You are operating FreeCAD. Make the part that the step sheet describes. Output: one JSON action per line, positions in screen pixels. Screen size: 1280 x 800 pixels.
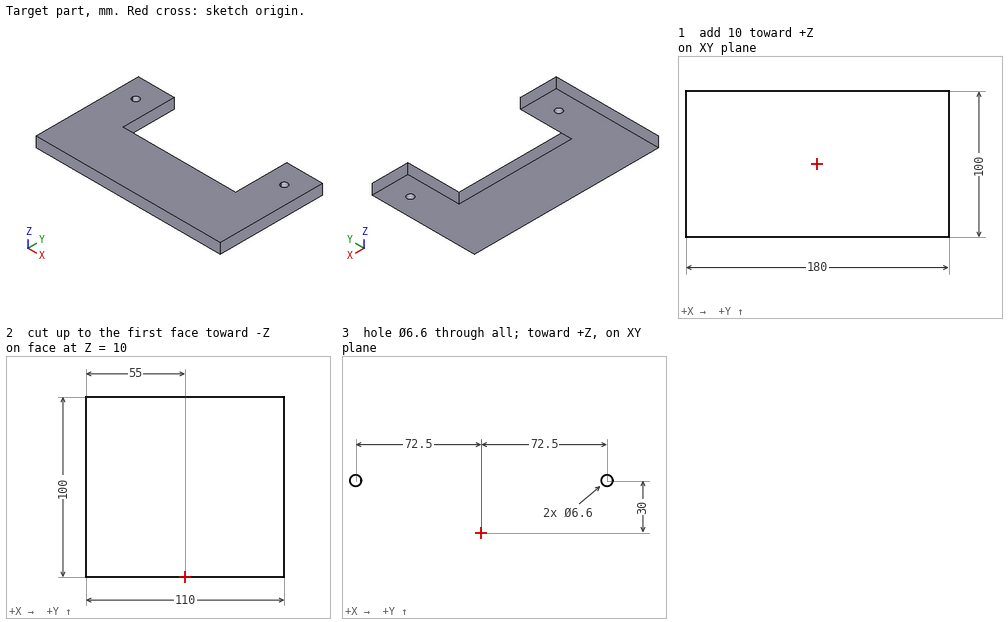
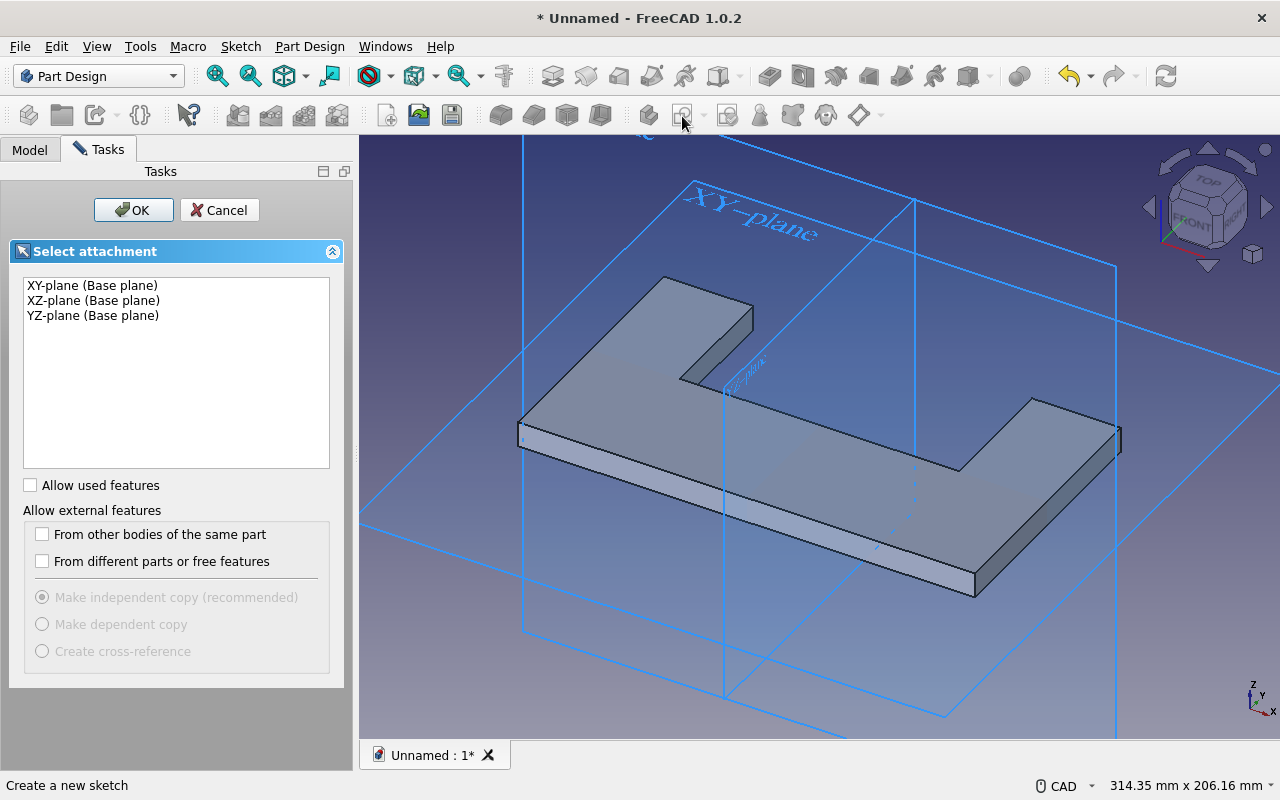
{"action": "left_click", "coordinate": [84, 286]}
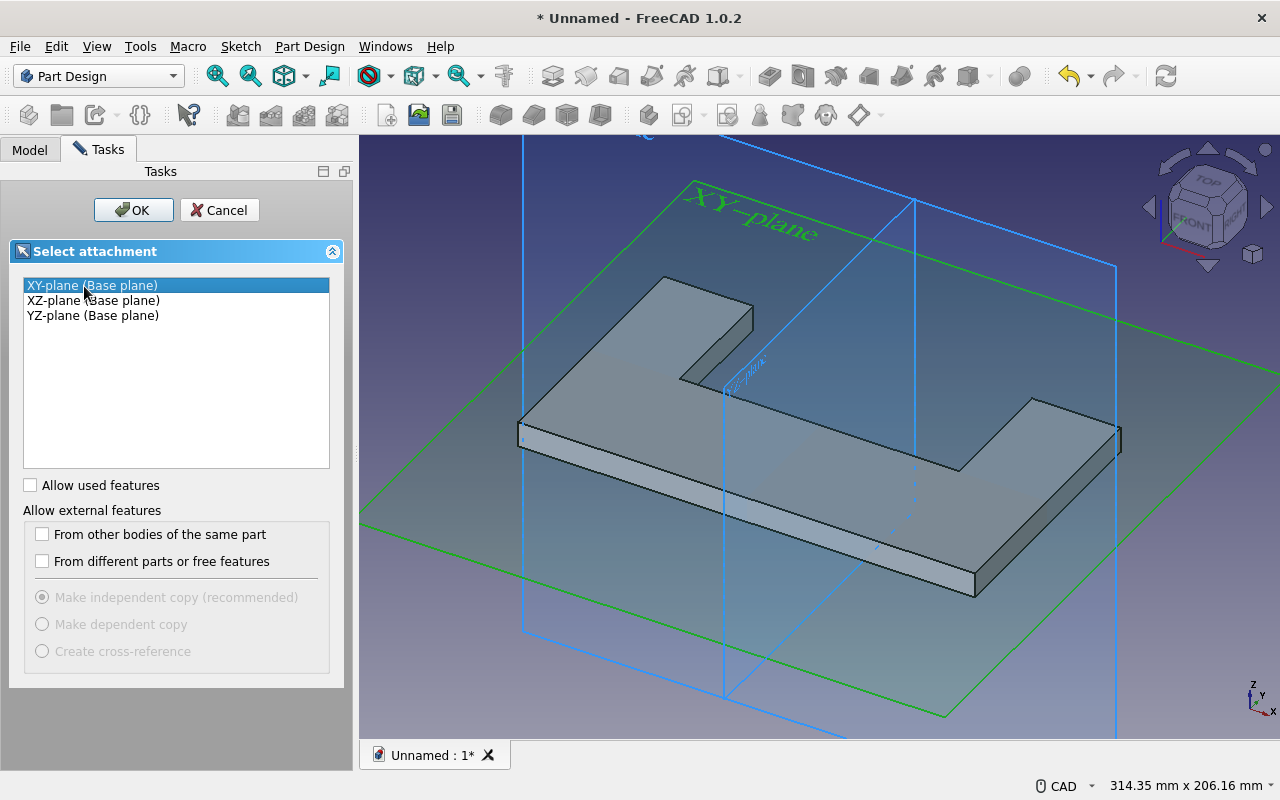
{"action": "left_click", "coordinate": [134, 210]}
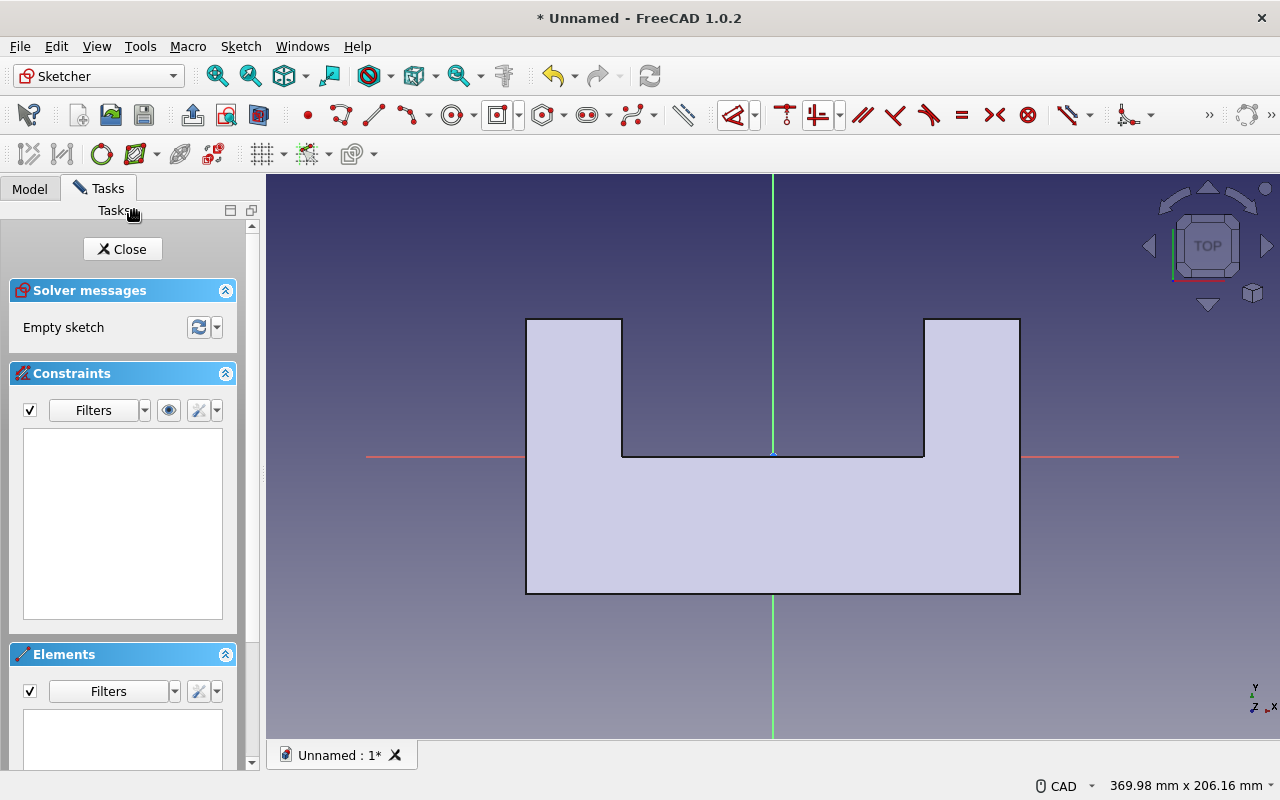
{"action": "left_click", "coordinate": [259, 116]}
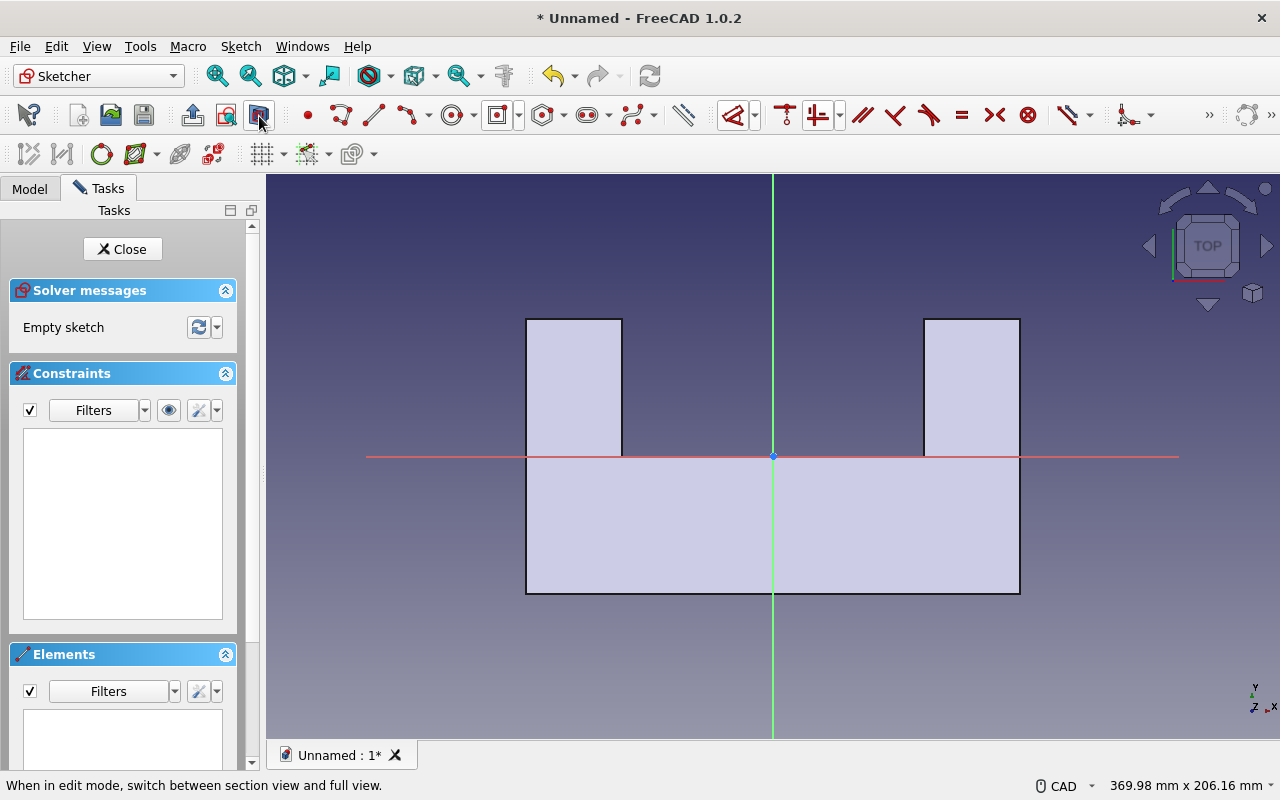
{"action": "scroll", "coordinate": [912, 318], "scroll_direction": "up", "scroll_amount": 2}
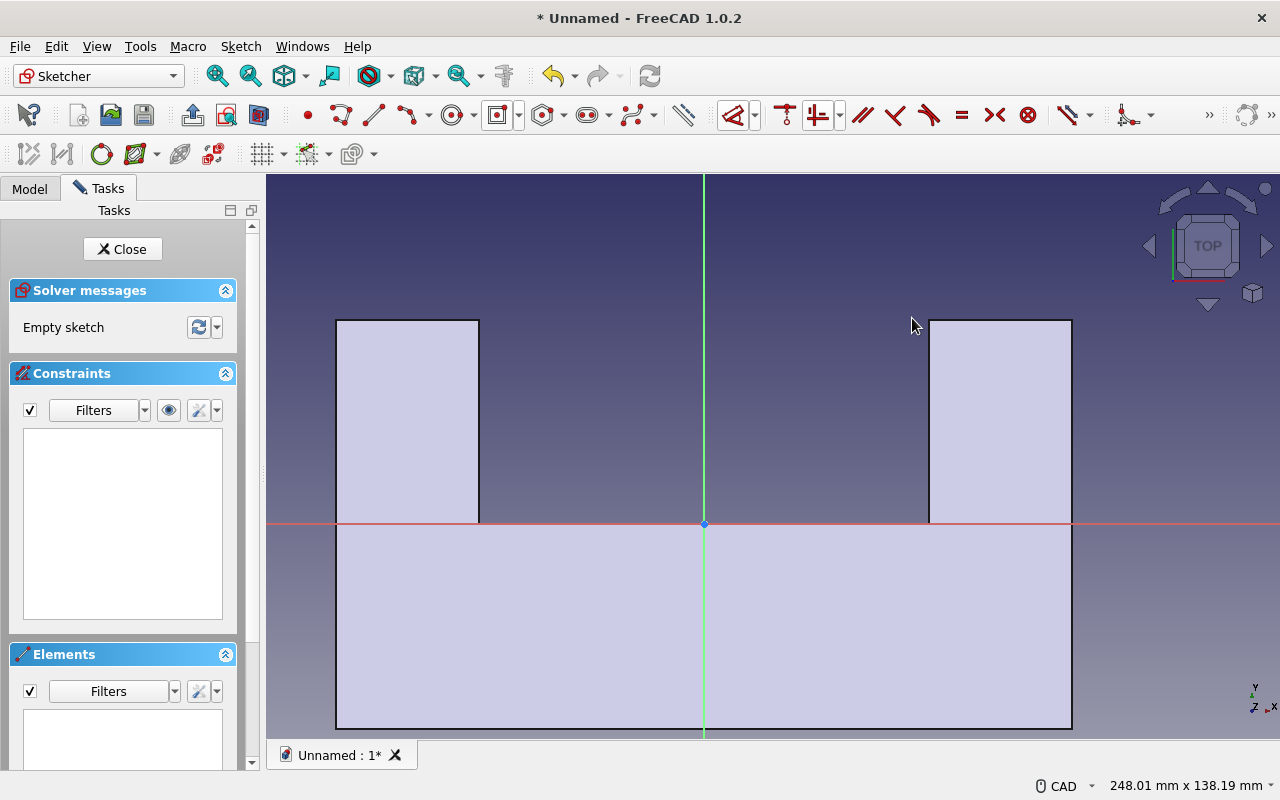
{"action": "left_click", "coordinate": [452, 116]}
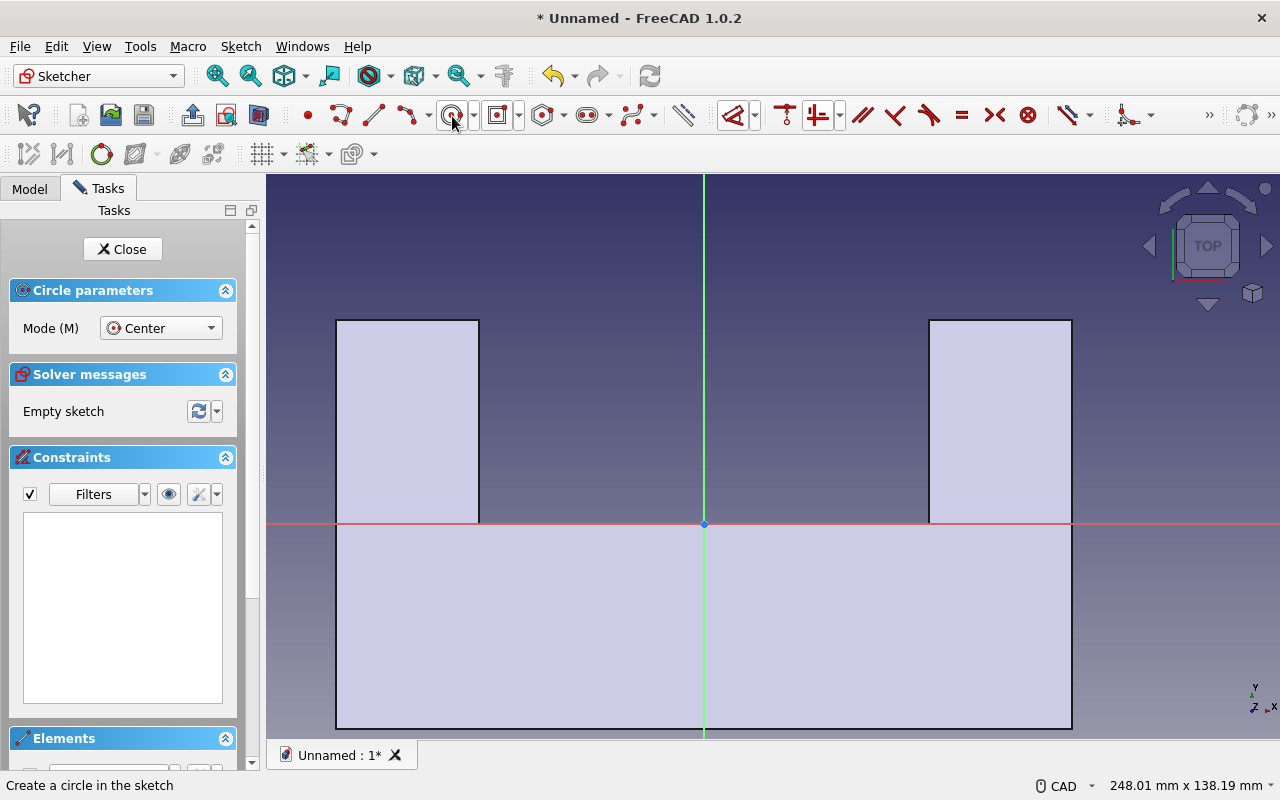
{"action": "scroll", "coordinate": [1001, 402], "scroll_direction": "up", "scroll_amount": 3}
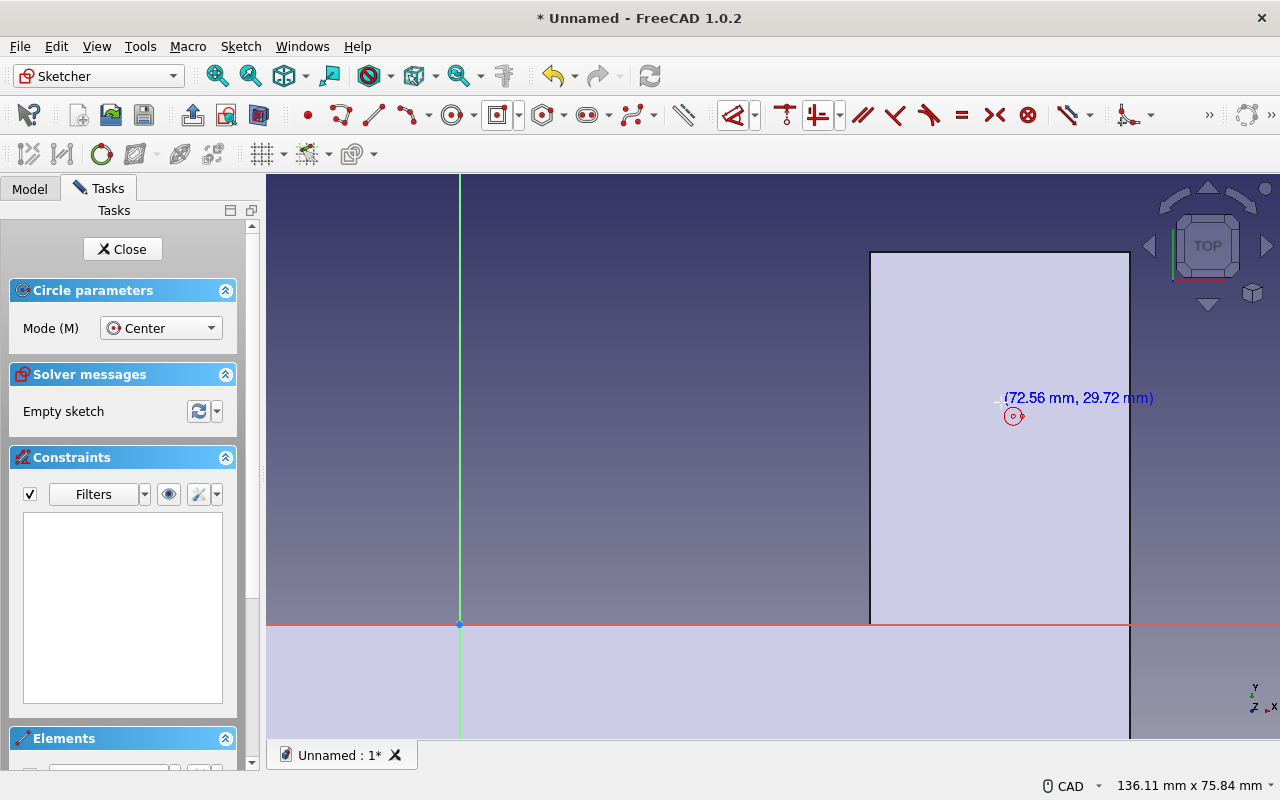
{"action": "left_click", "coordinate": [1000, 401]}
{"action": "left_click", "coordinate": [1017, 384]}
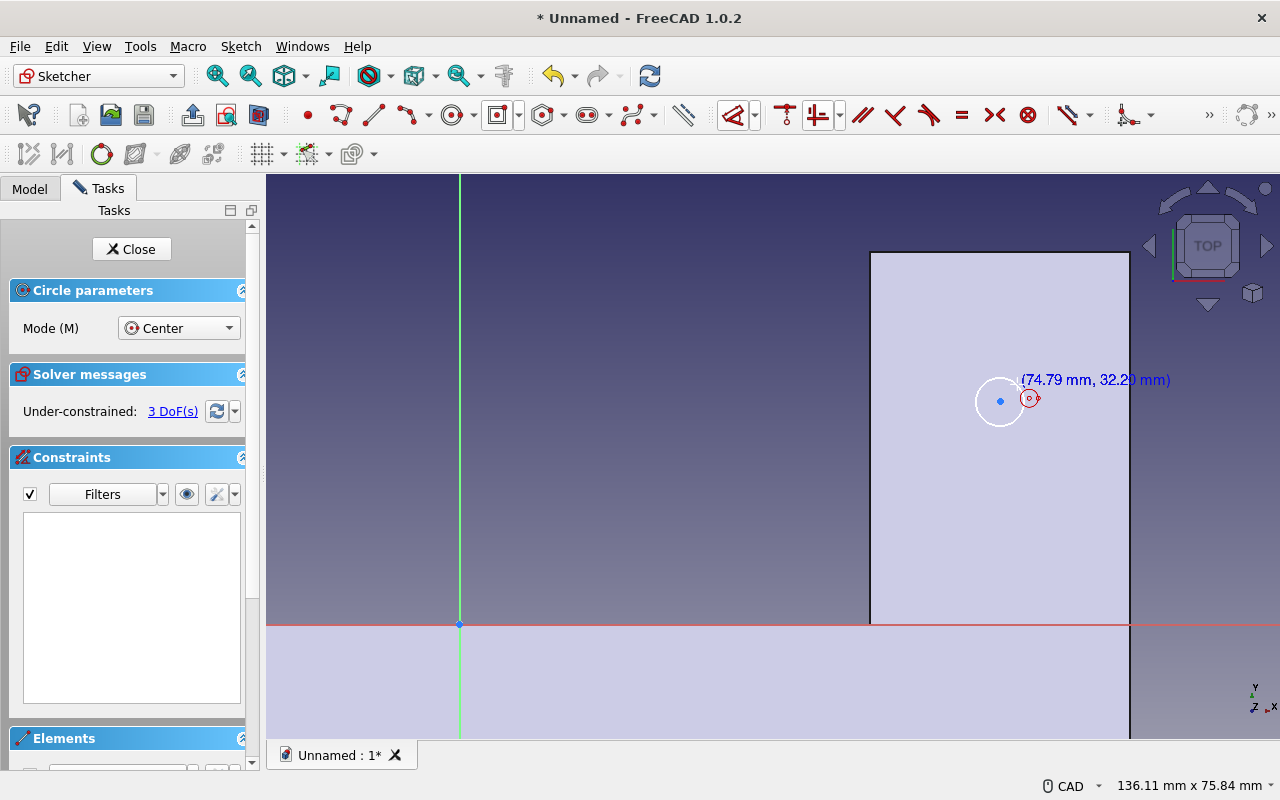
{"action": "scroll", "coordinate": [1002, 403], "scroll_direction": "down", "scroll_amount": 3}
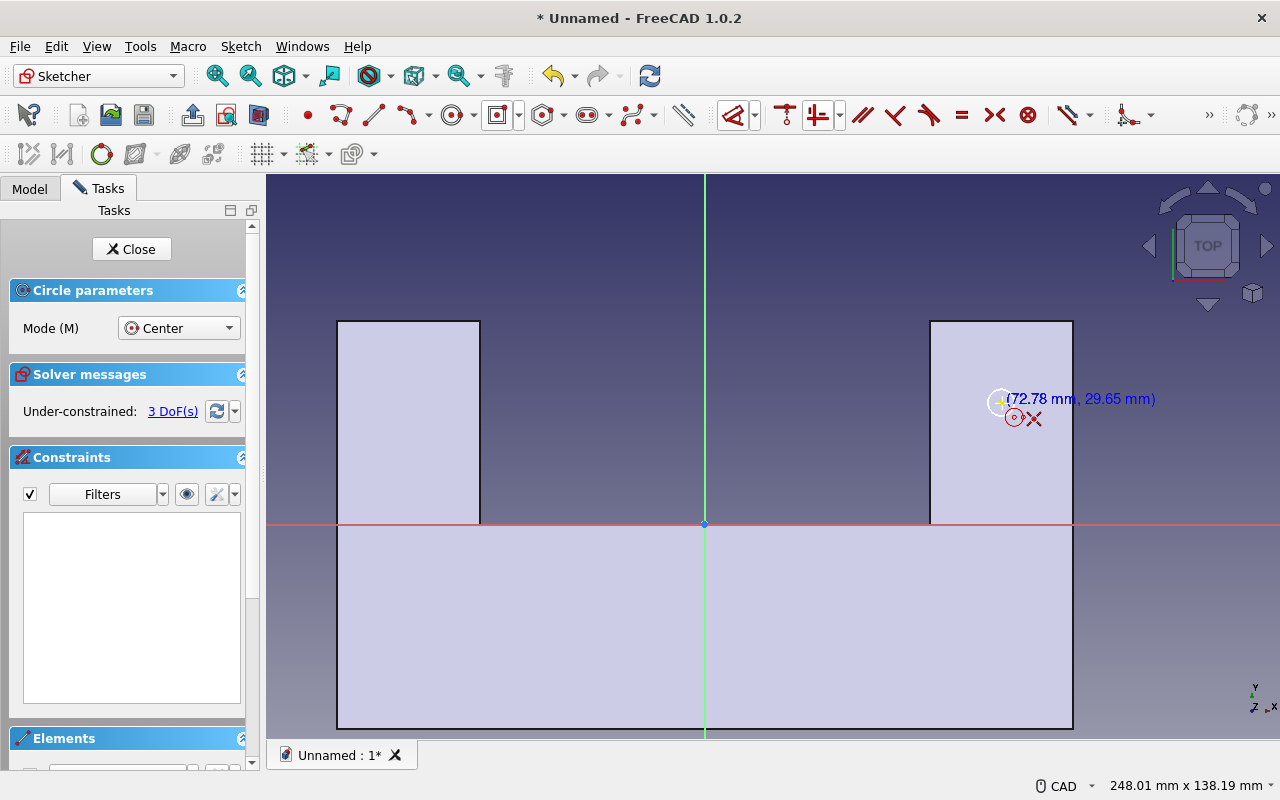
{"action": "scroll", "coordinate": [408, 402], "scroll_direction": "up", "scroll_amount": 3}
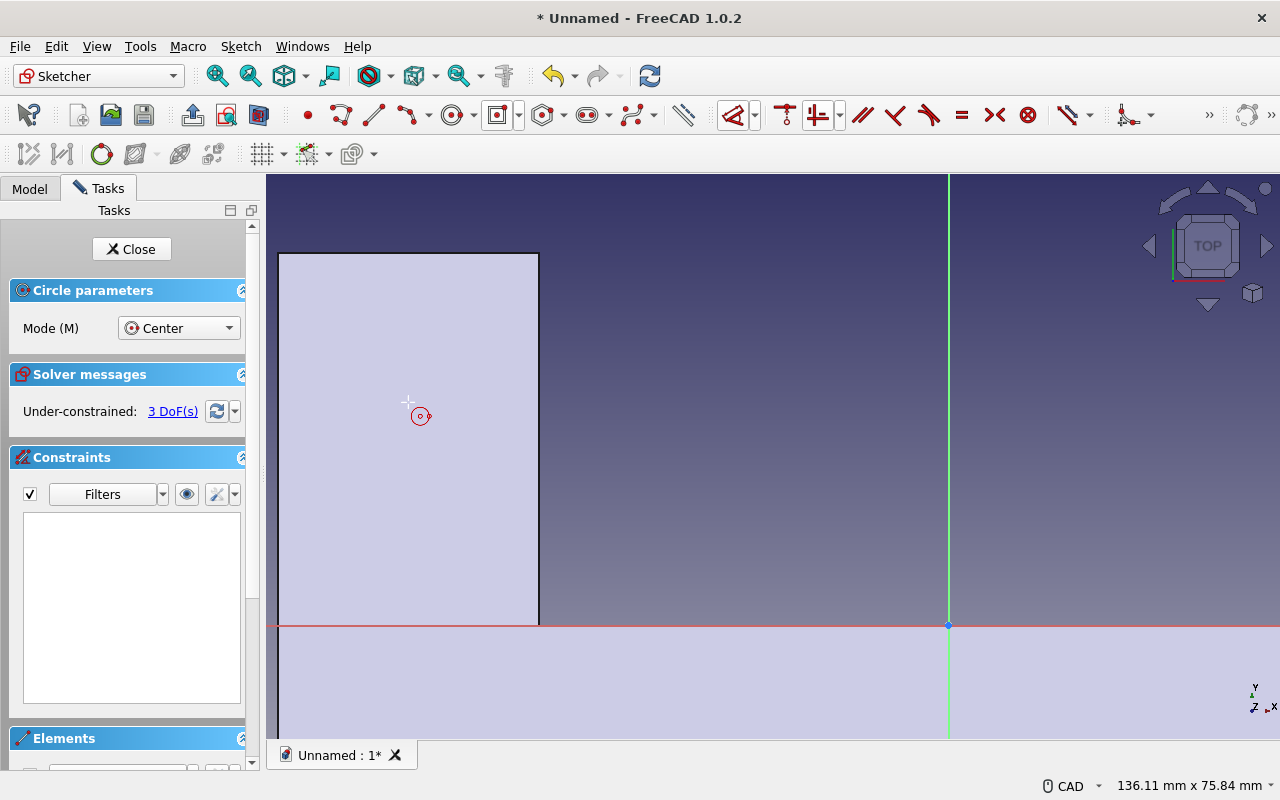
{"action": "left_click", "coordinate": [409, 402]}
{"action": "left_click", "coordinate": [426, 385]}
{"action": "key", "text": "Escape"}